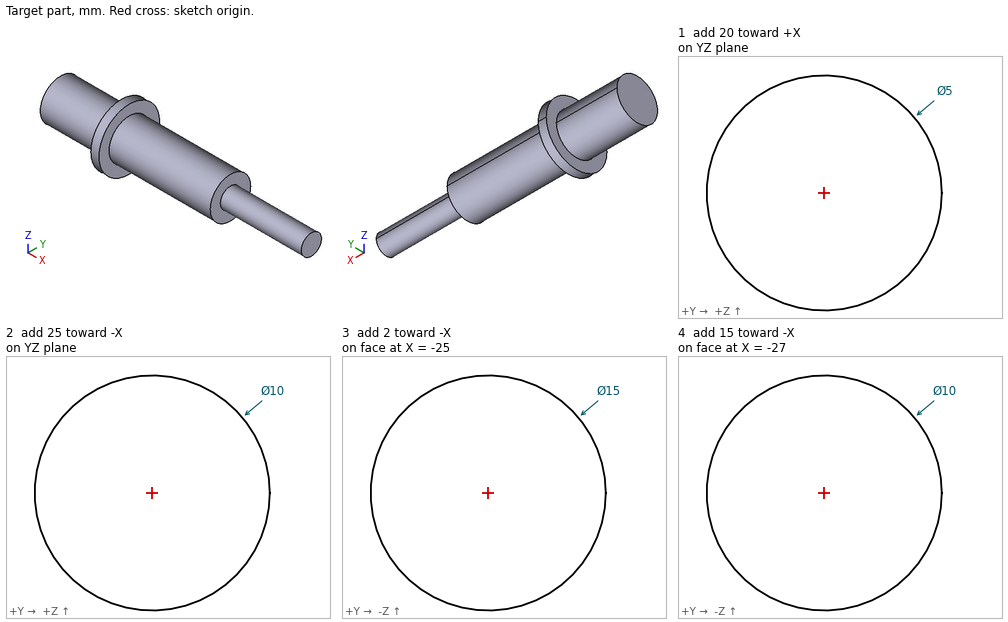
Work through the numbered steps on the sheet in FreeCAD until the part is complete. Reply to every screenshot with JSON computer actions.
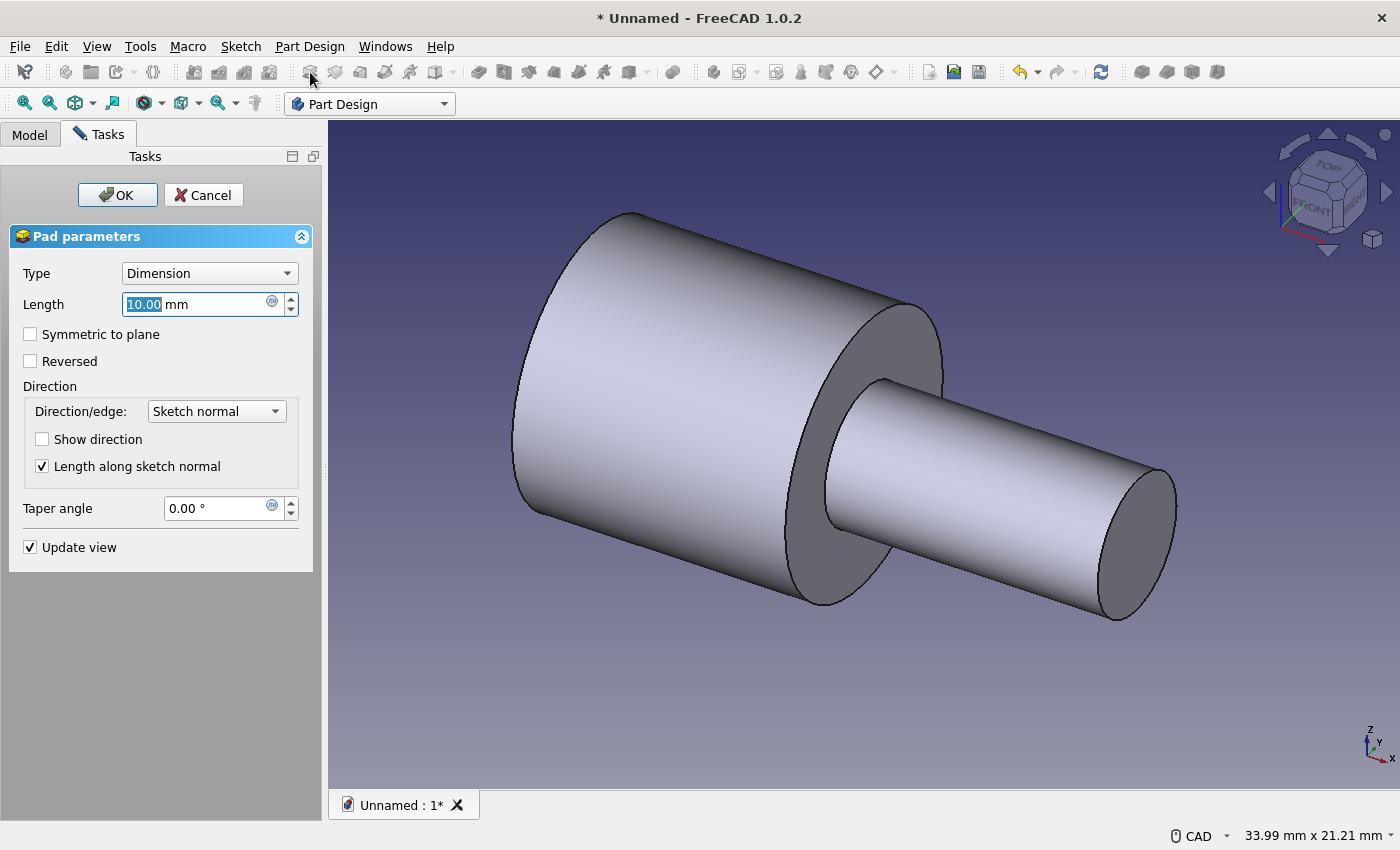
{"action": "type", "text": "25"}
{"action": "key", "text": "Tab"}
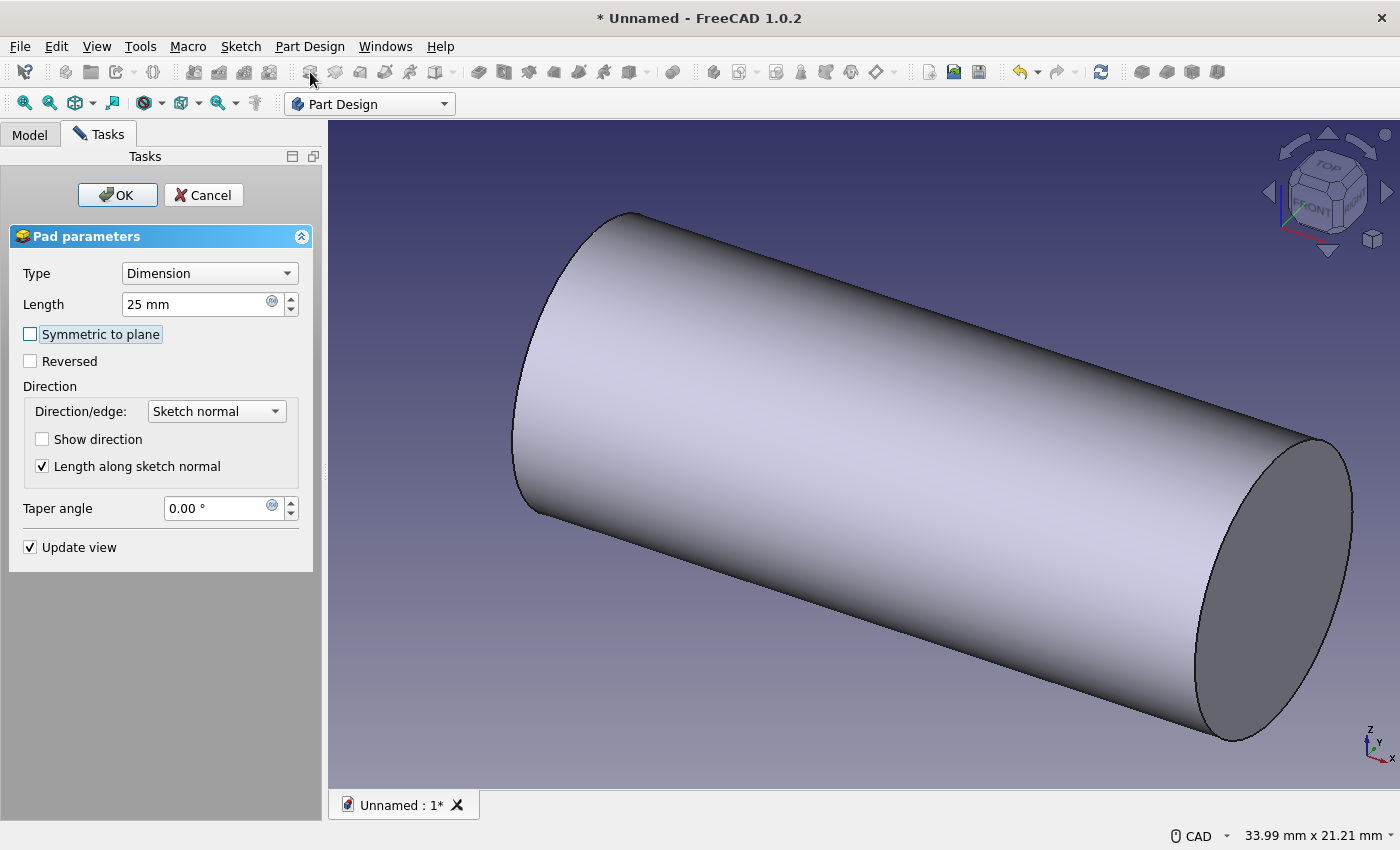
{"action": "left_click", "coordinate": [31, 361]}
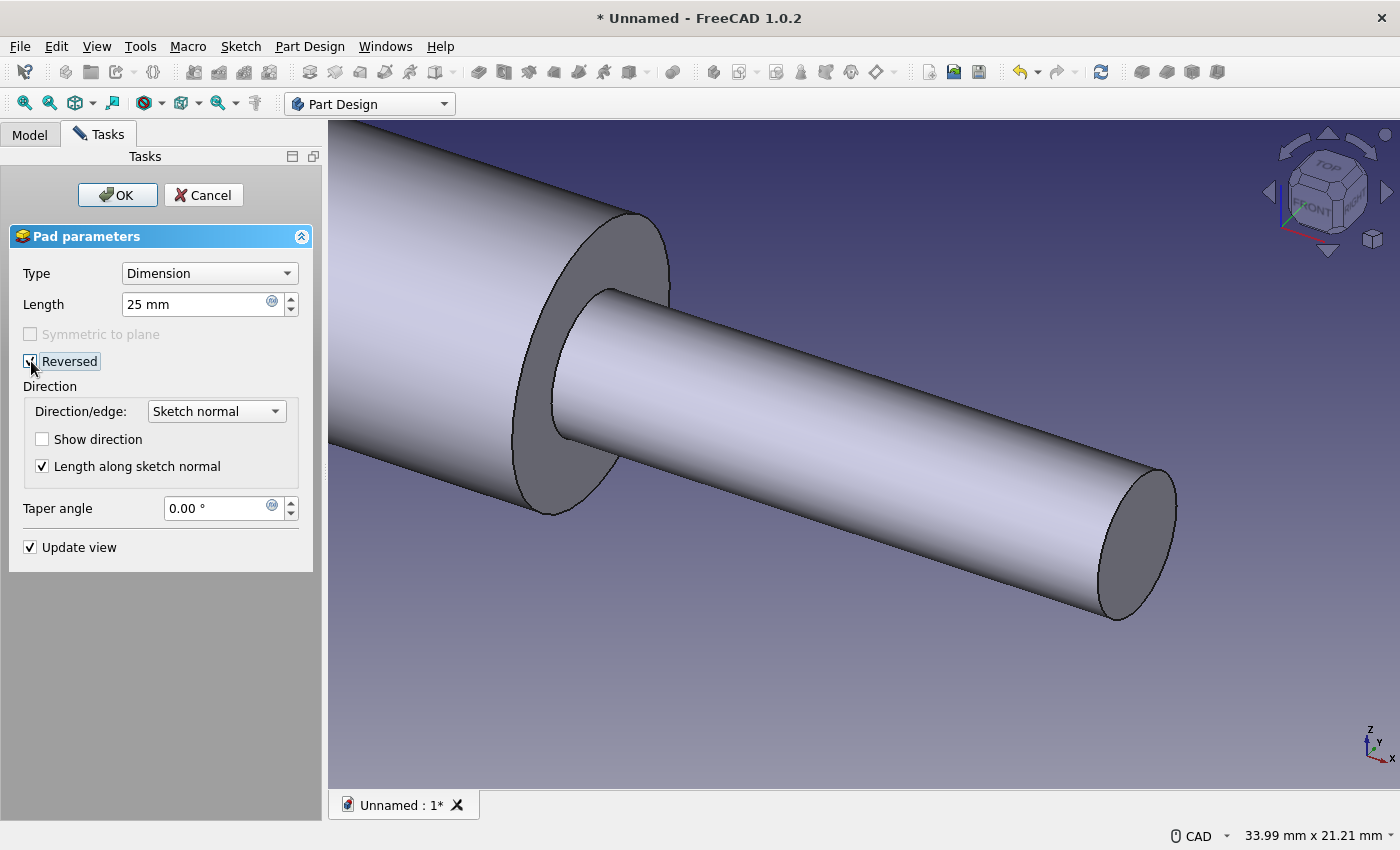
{"action": "left_click", "coordinate": [118, 195]}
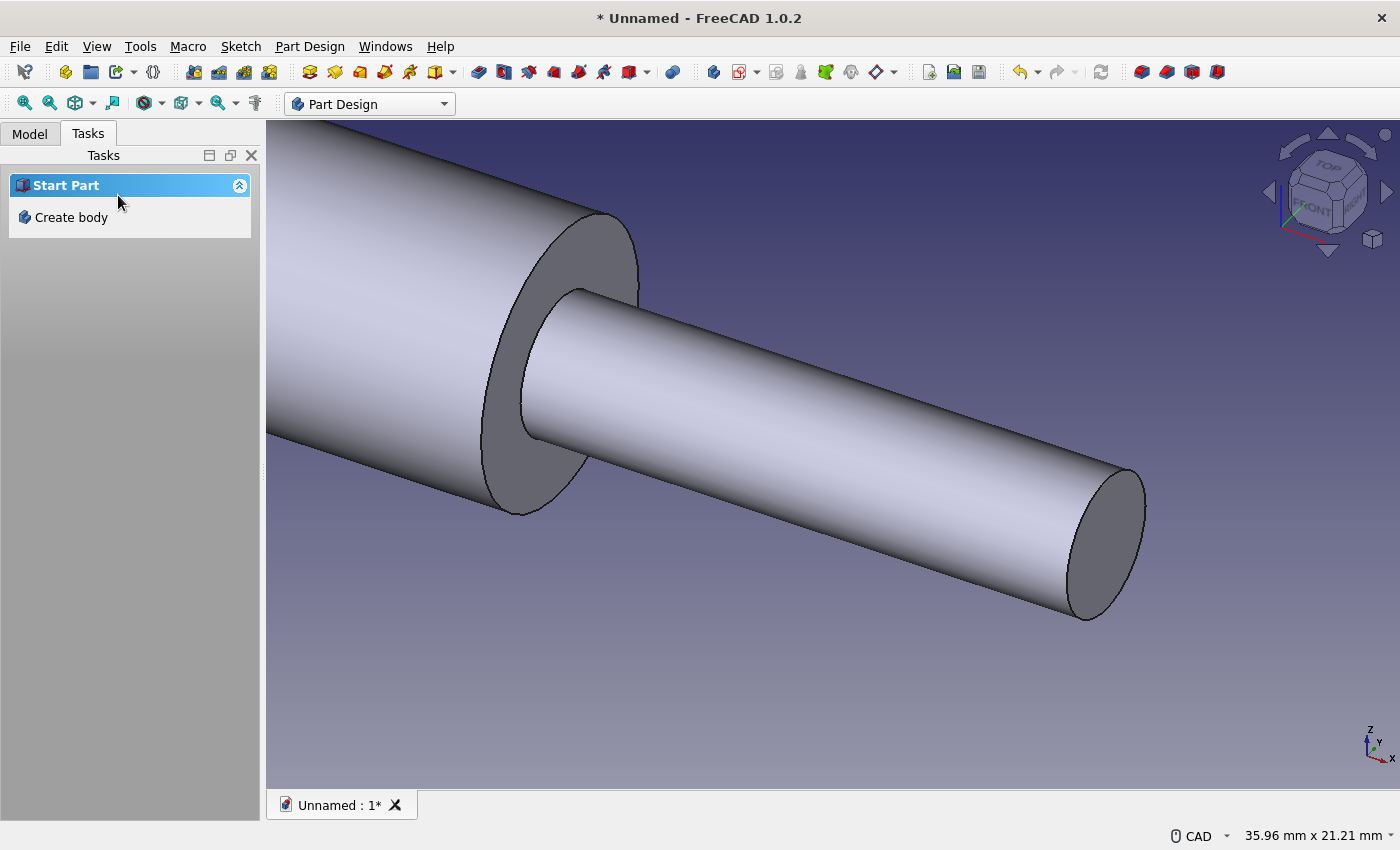
{"action": "key", "text": "v f"}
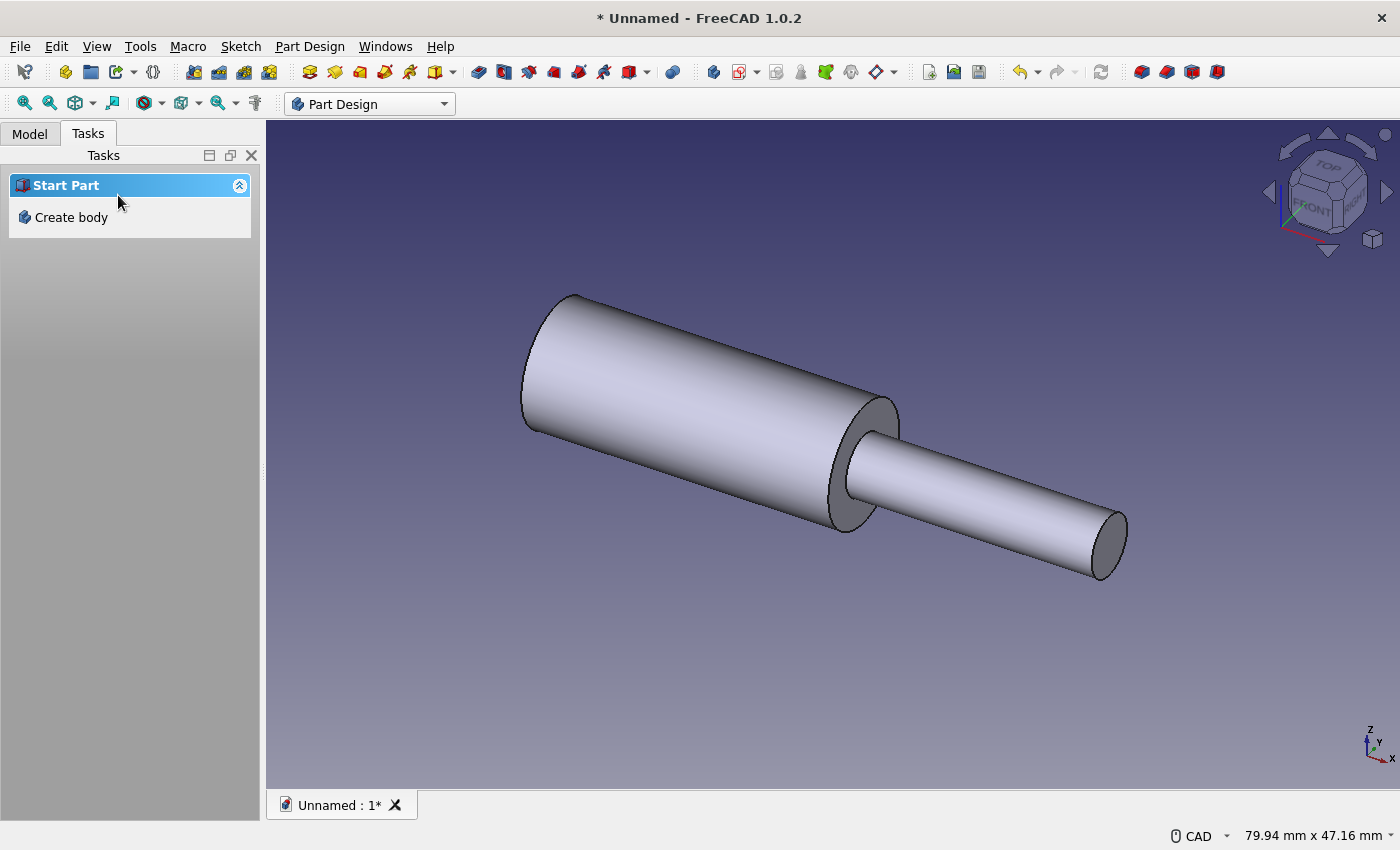
{"action": "key", "text": "6"}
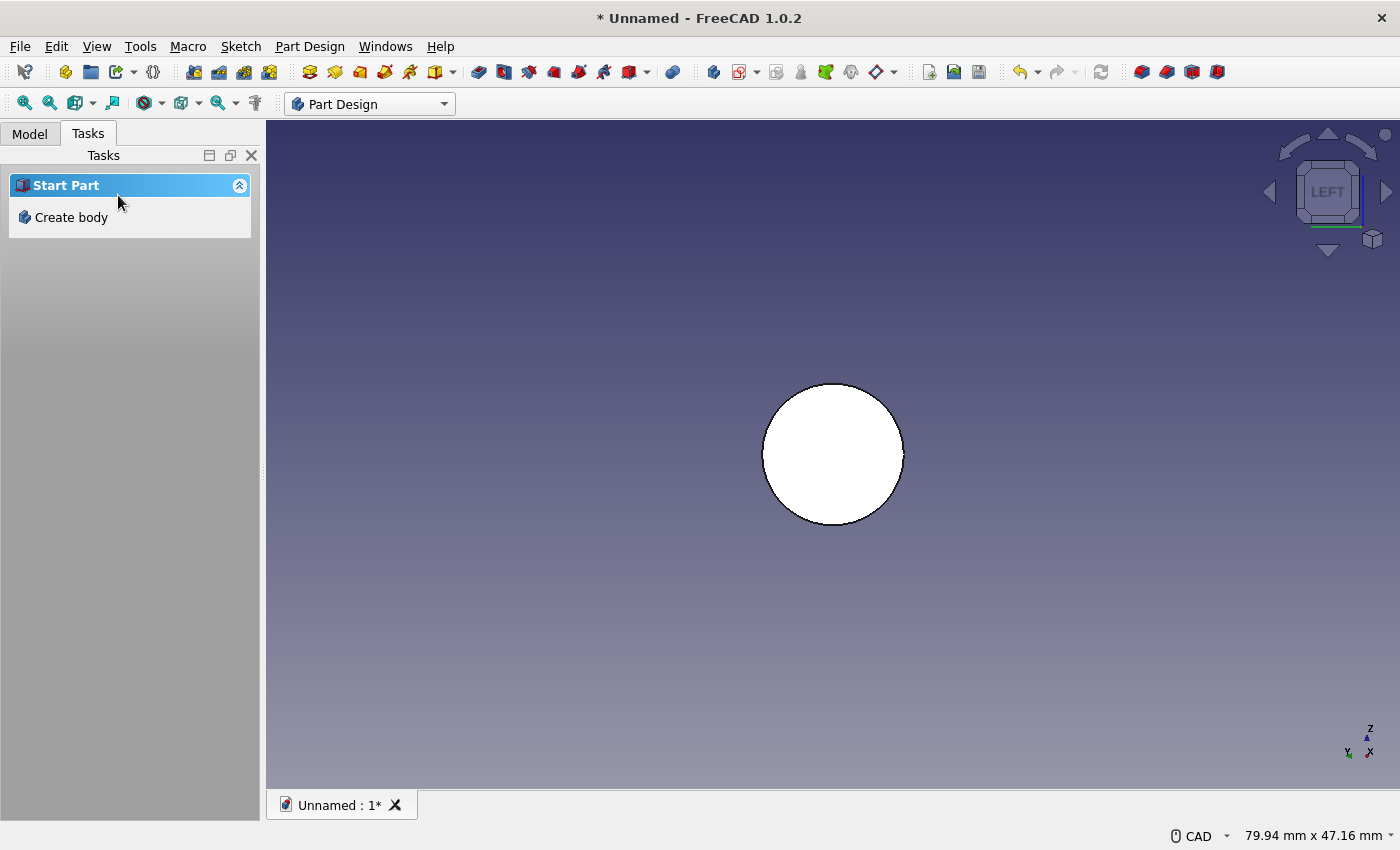
{"action": "key", "text": "v f"}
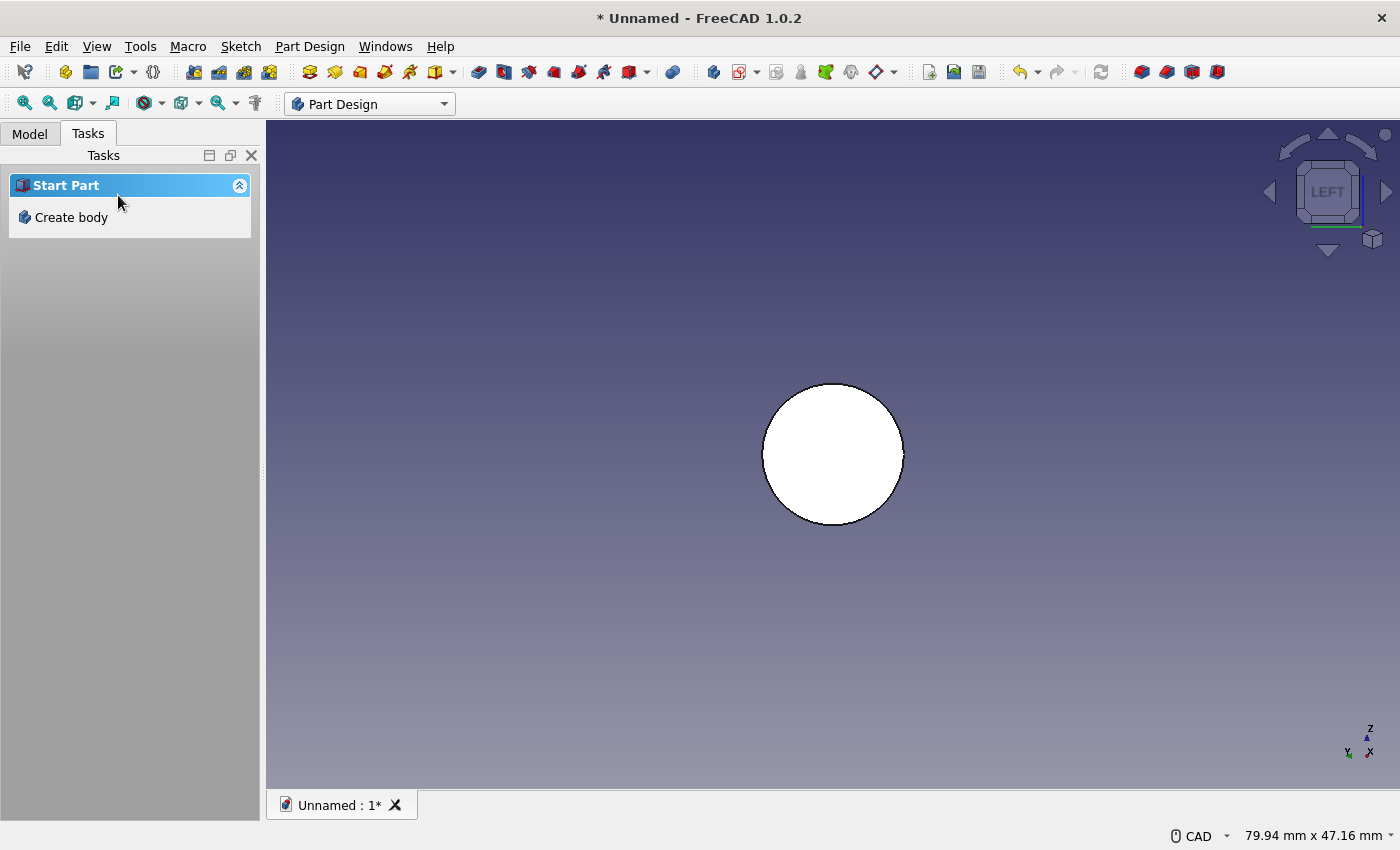
{"action": "left_click", "coordinate": [833, 453]}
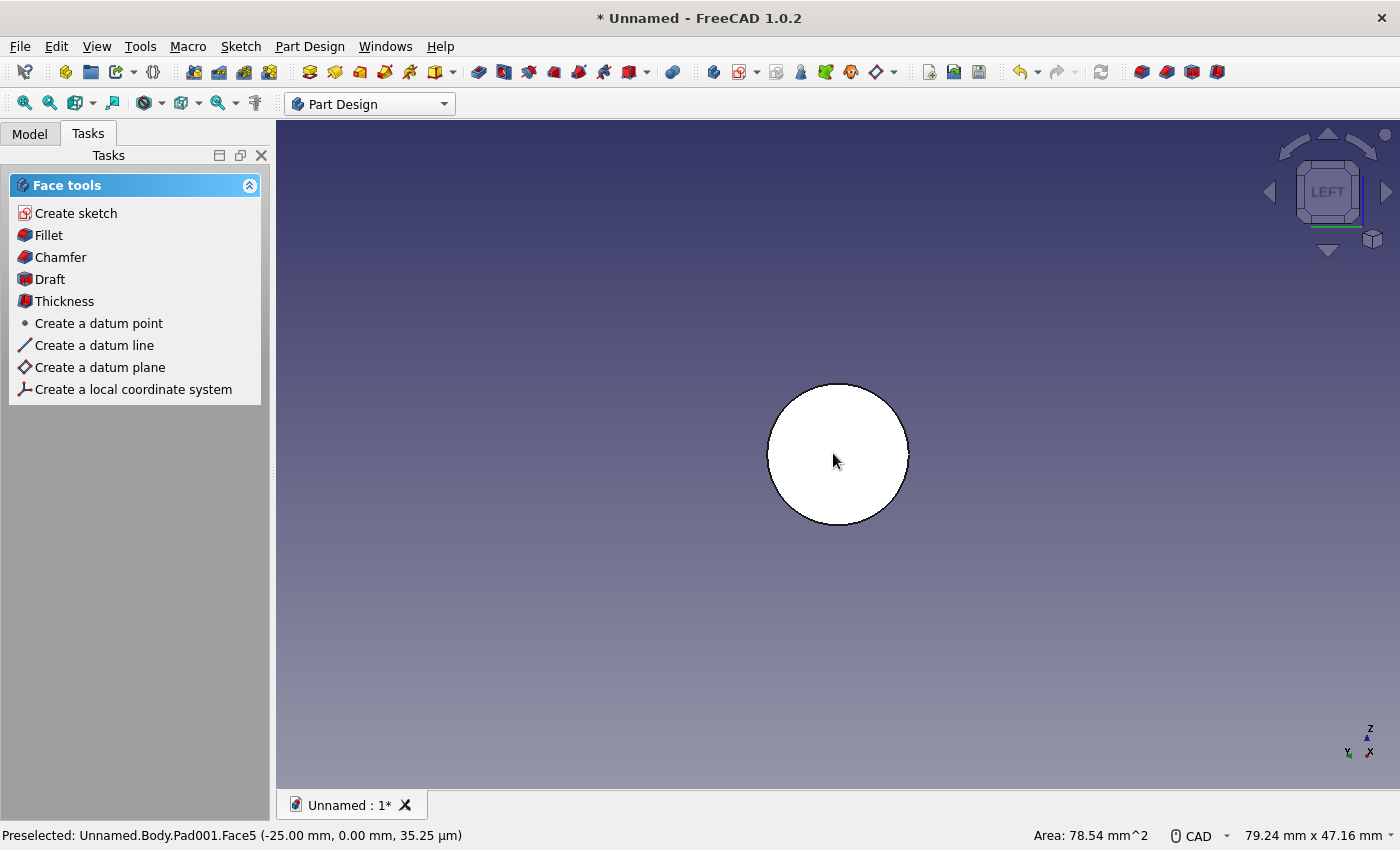
{"action": "left_click", "coordinate": [738, 72]}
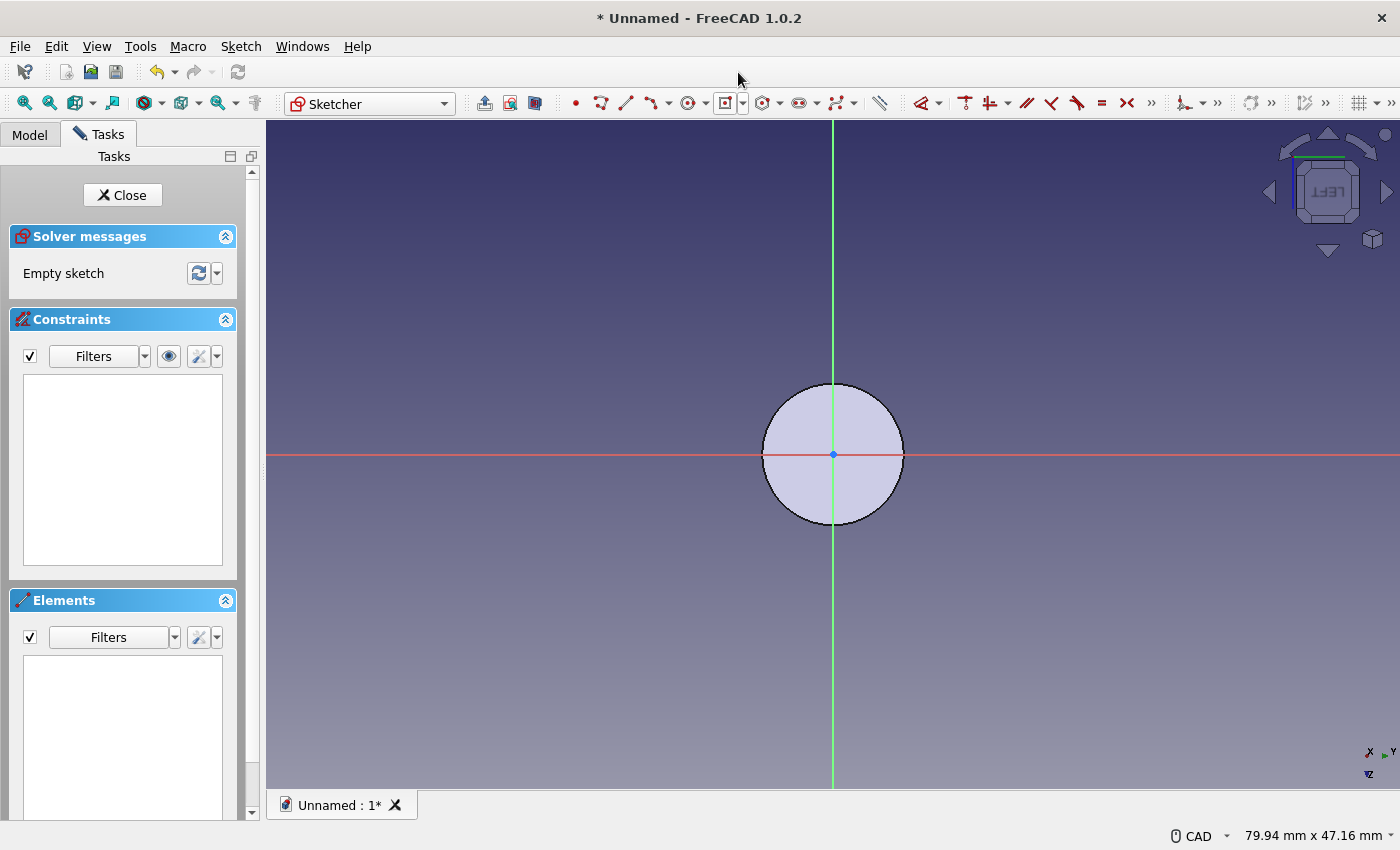
{"action": "scroll", "coordinate": [889, 455], "scroll_direction": "up", "scroll_amount": 4}